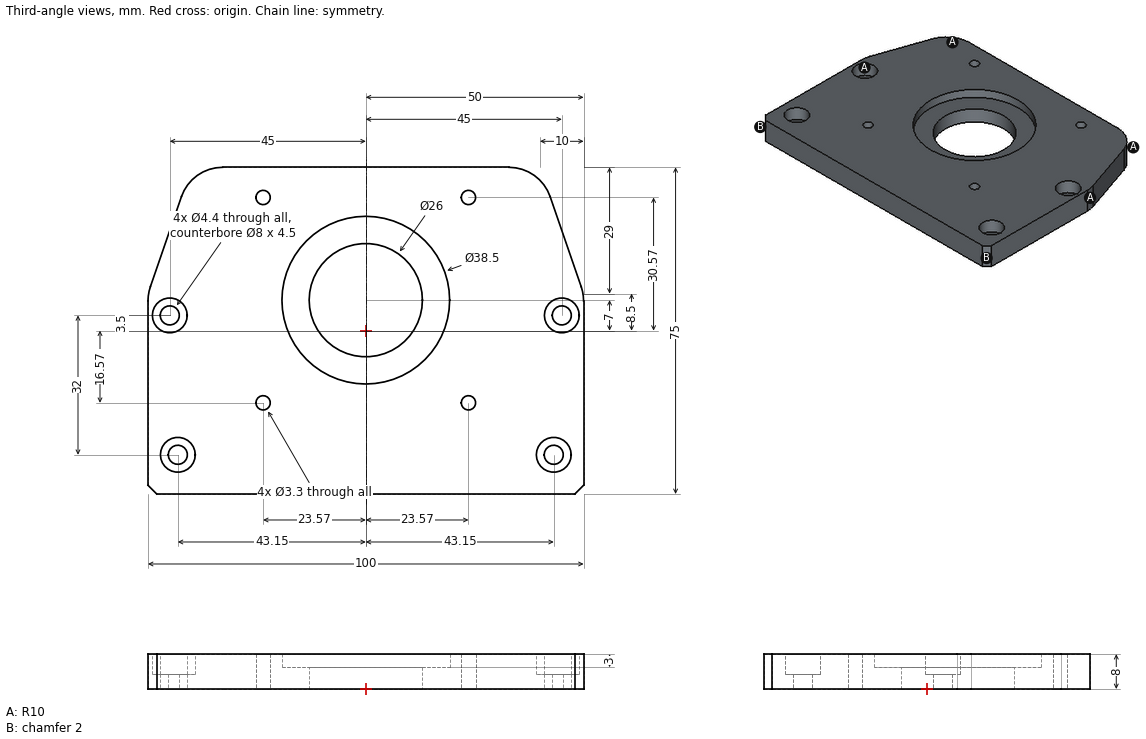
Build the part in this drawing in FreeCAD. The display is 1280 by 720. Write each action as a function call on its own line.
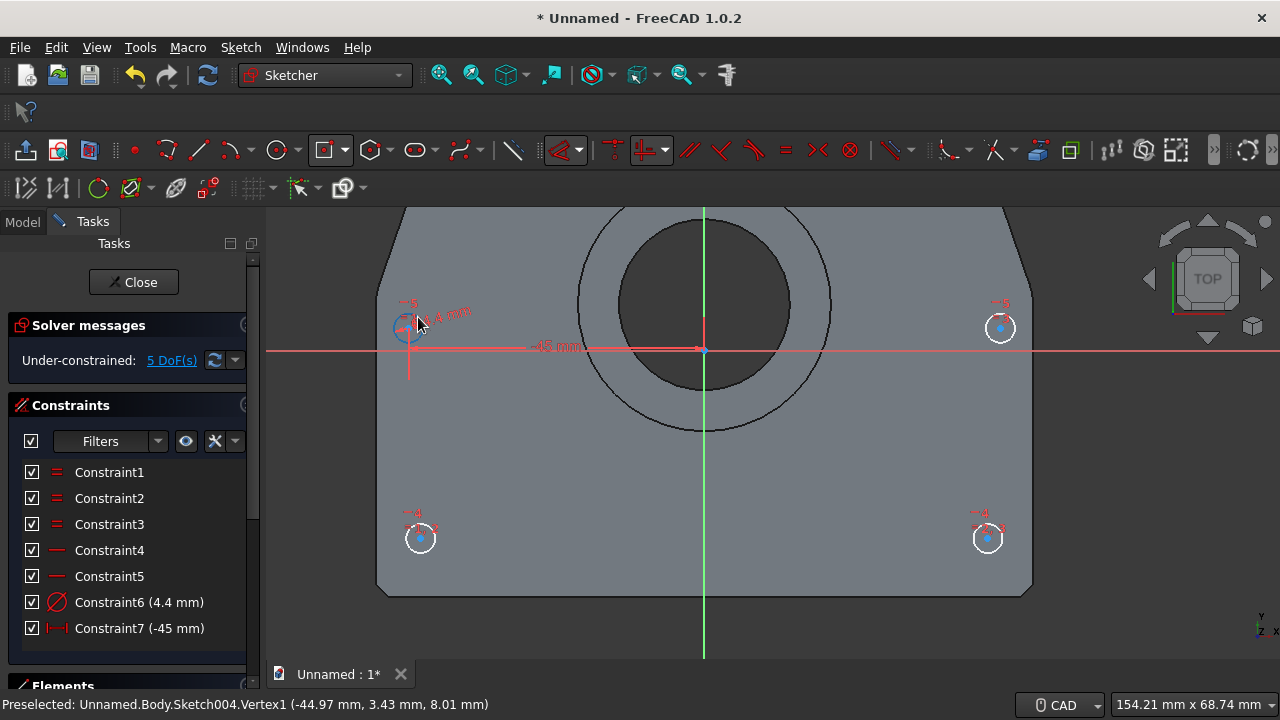
click(1000, 328)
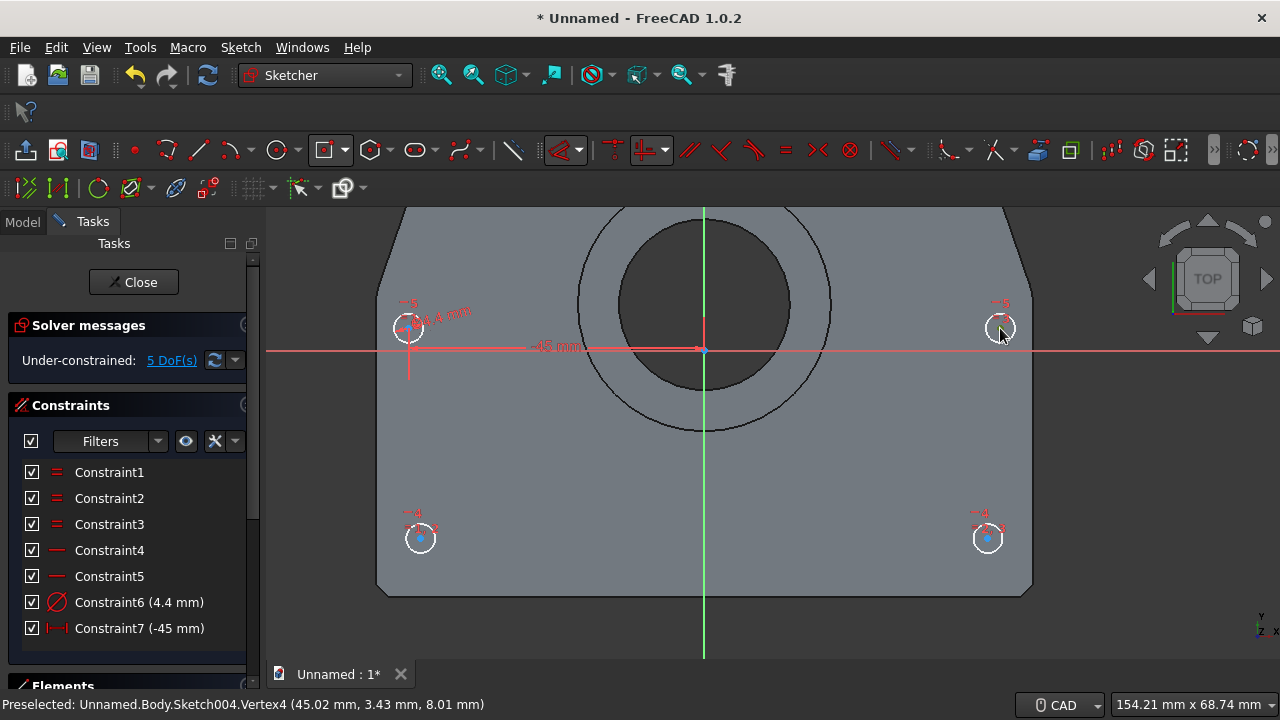
click(582, 150)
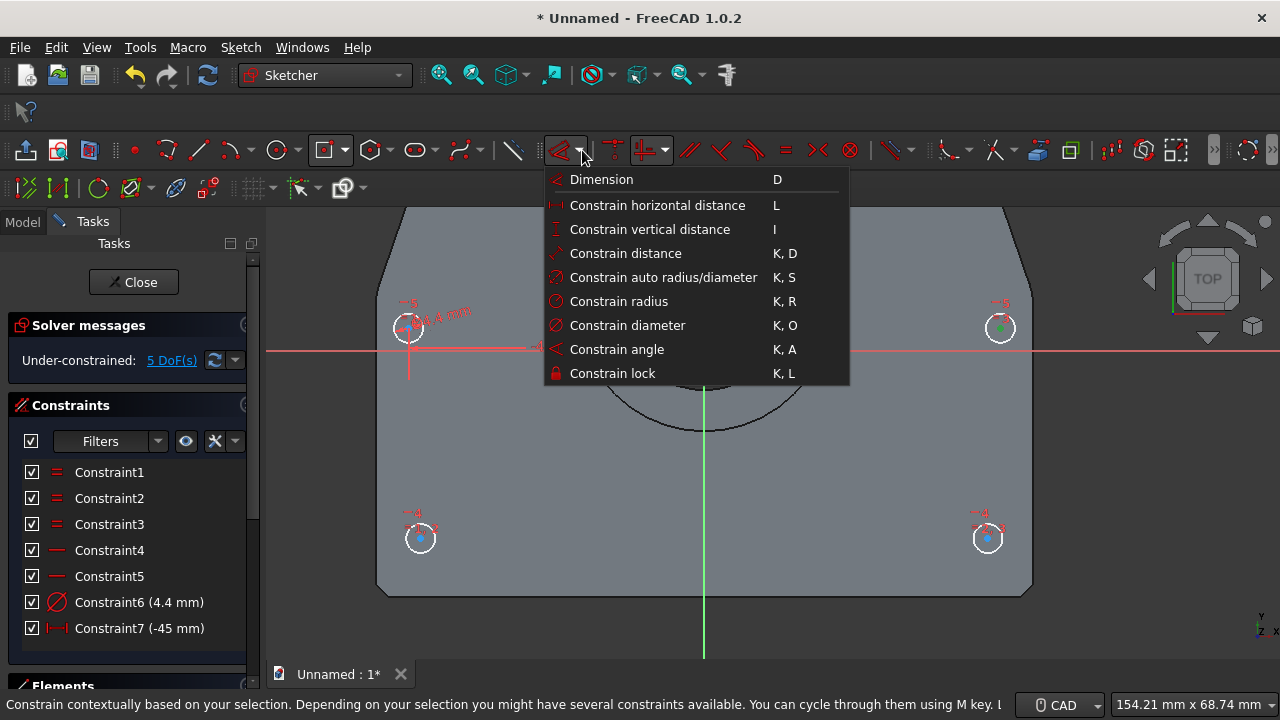
click(697, 205)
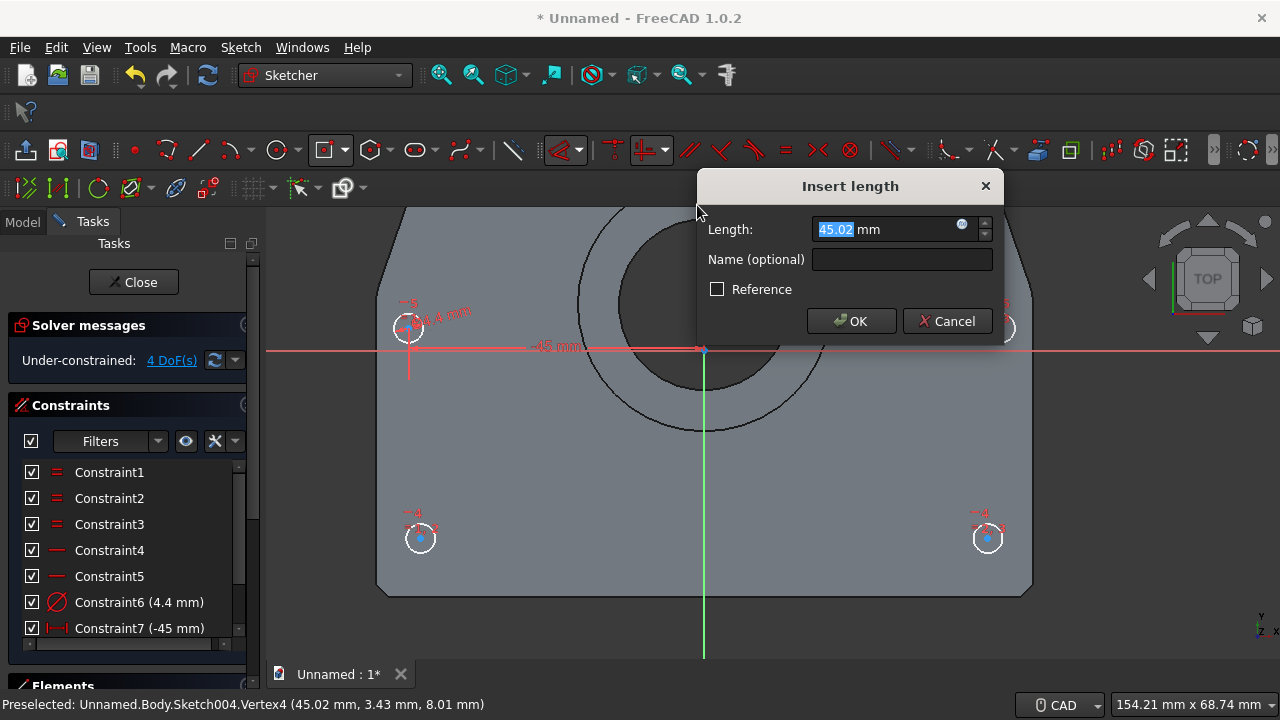
text(45)
key(Return)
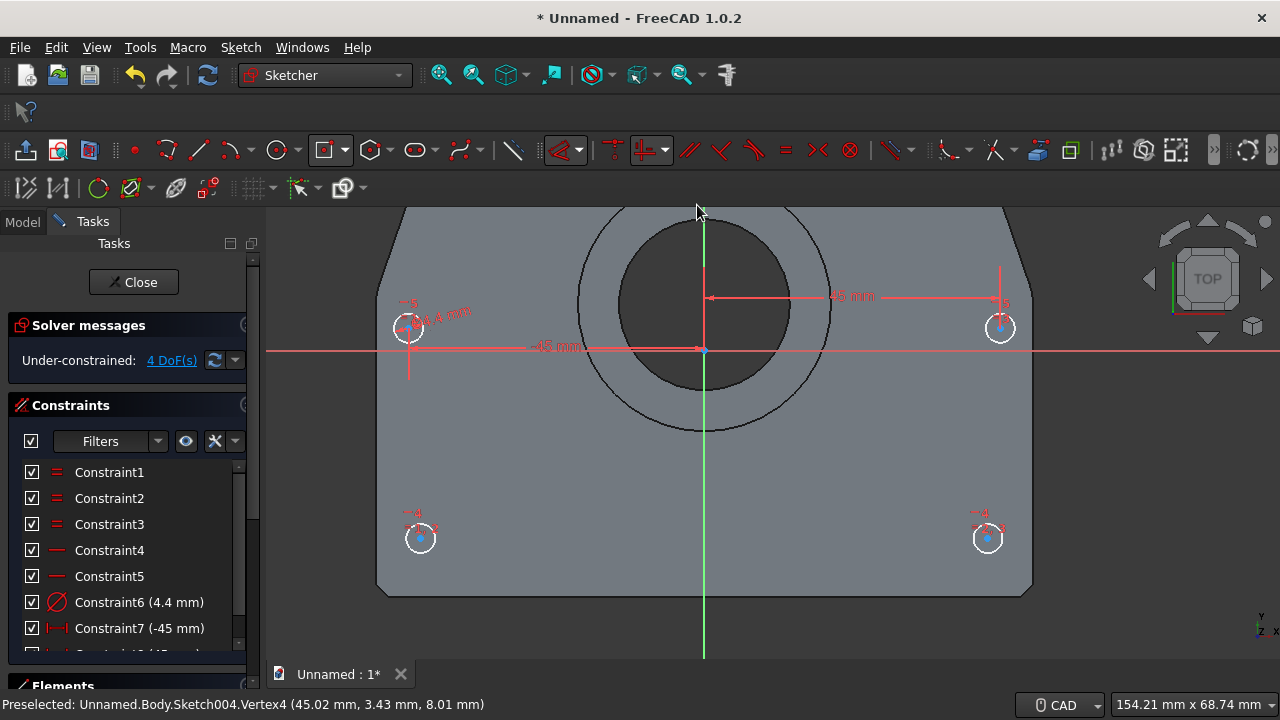
scroll(409, 328, up, 3)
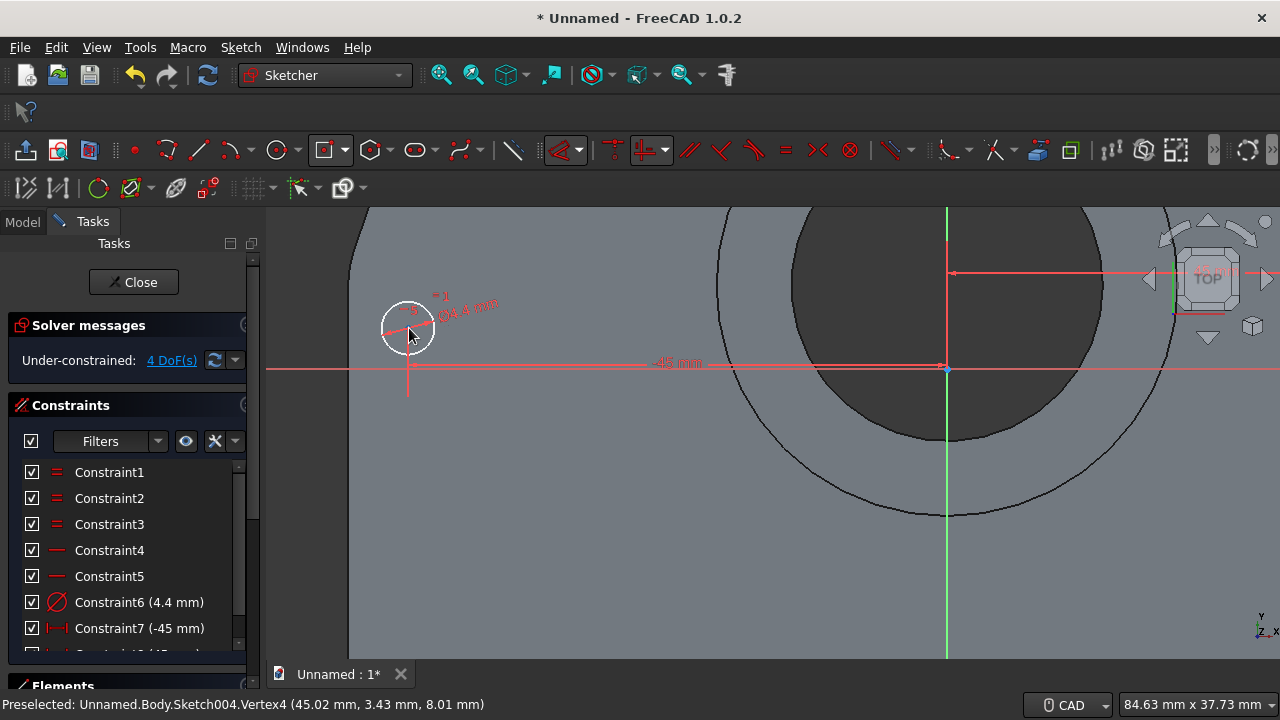
click(408, 328)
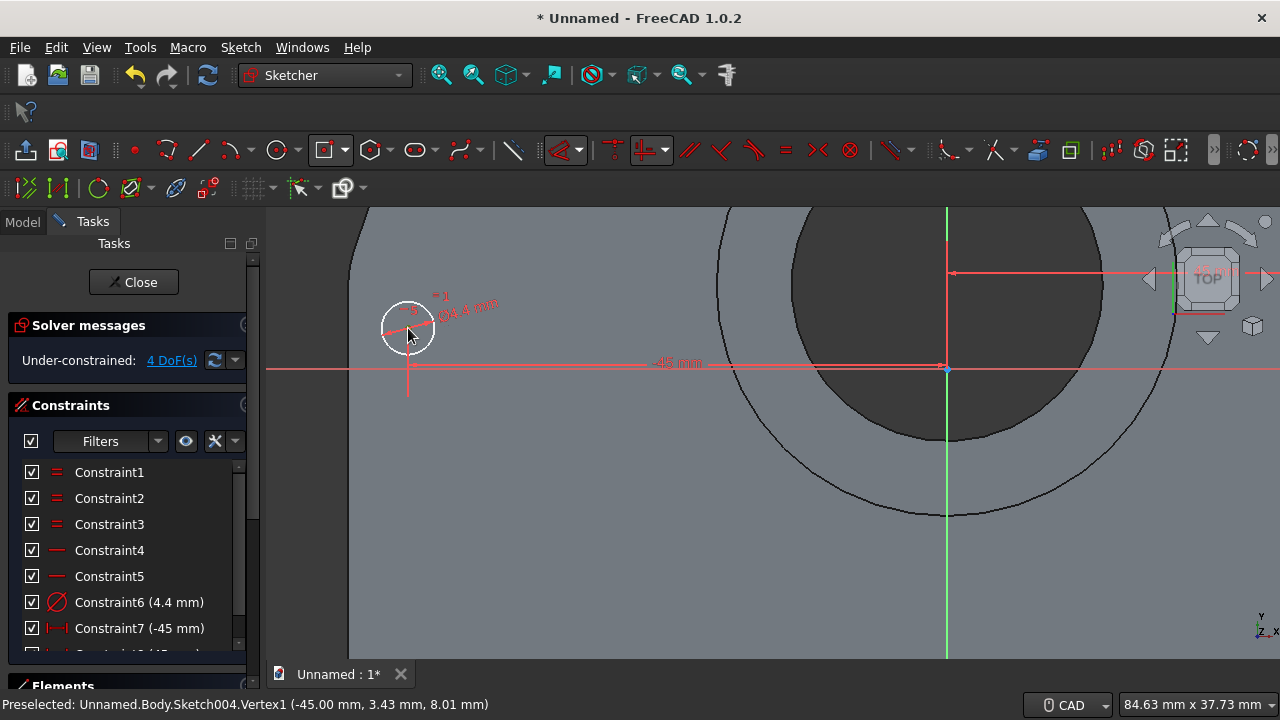
click(582, 150)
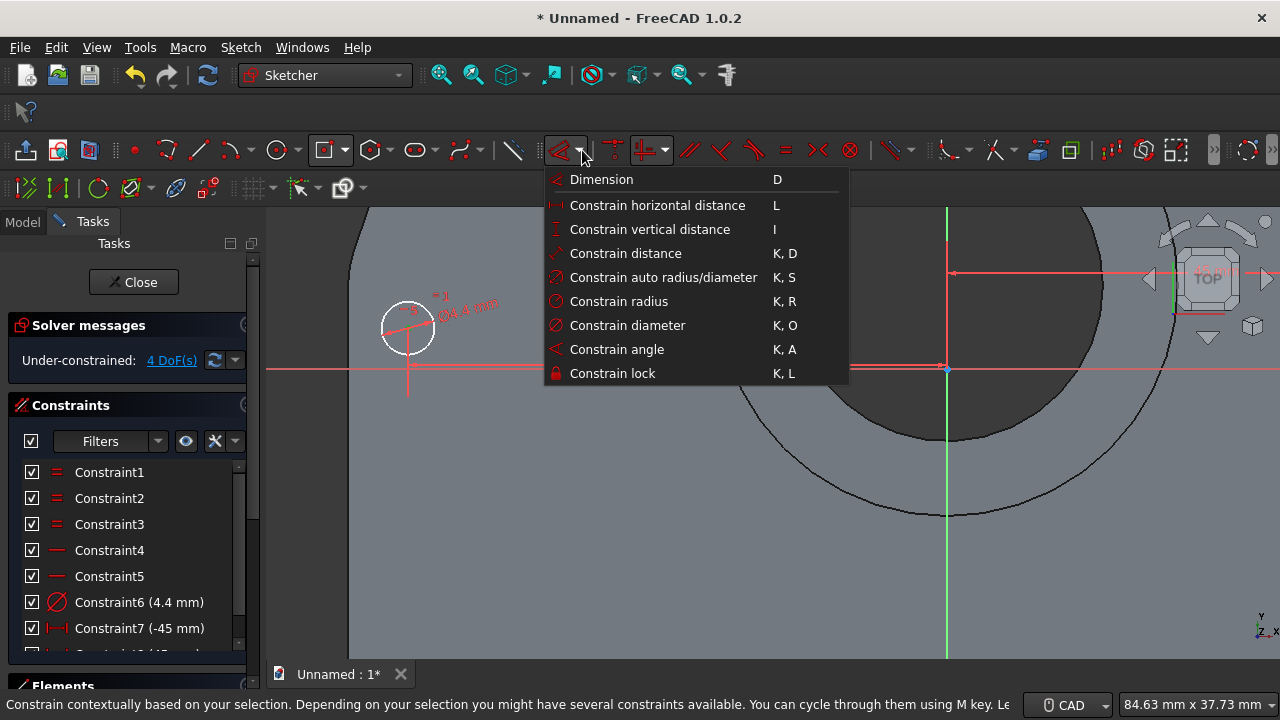
click(697, 229)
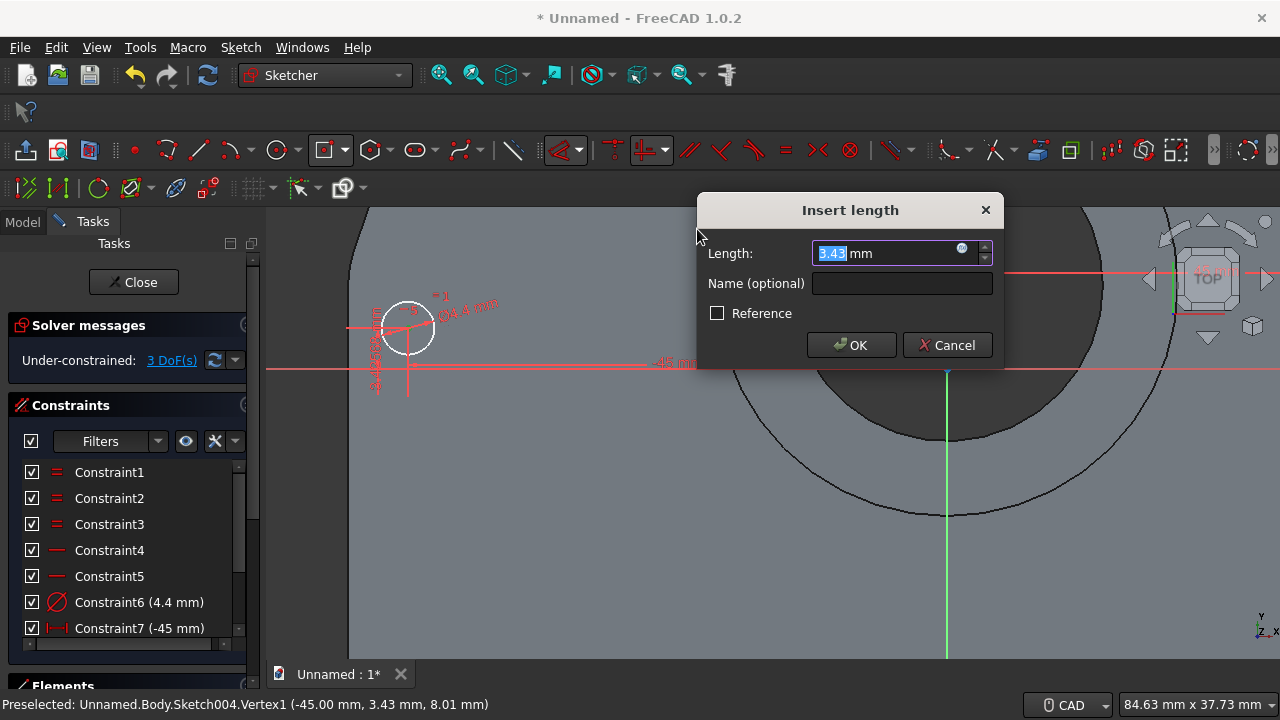
text(3.5)
key(Return)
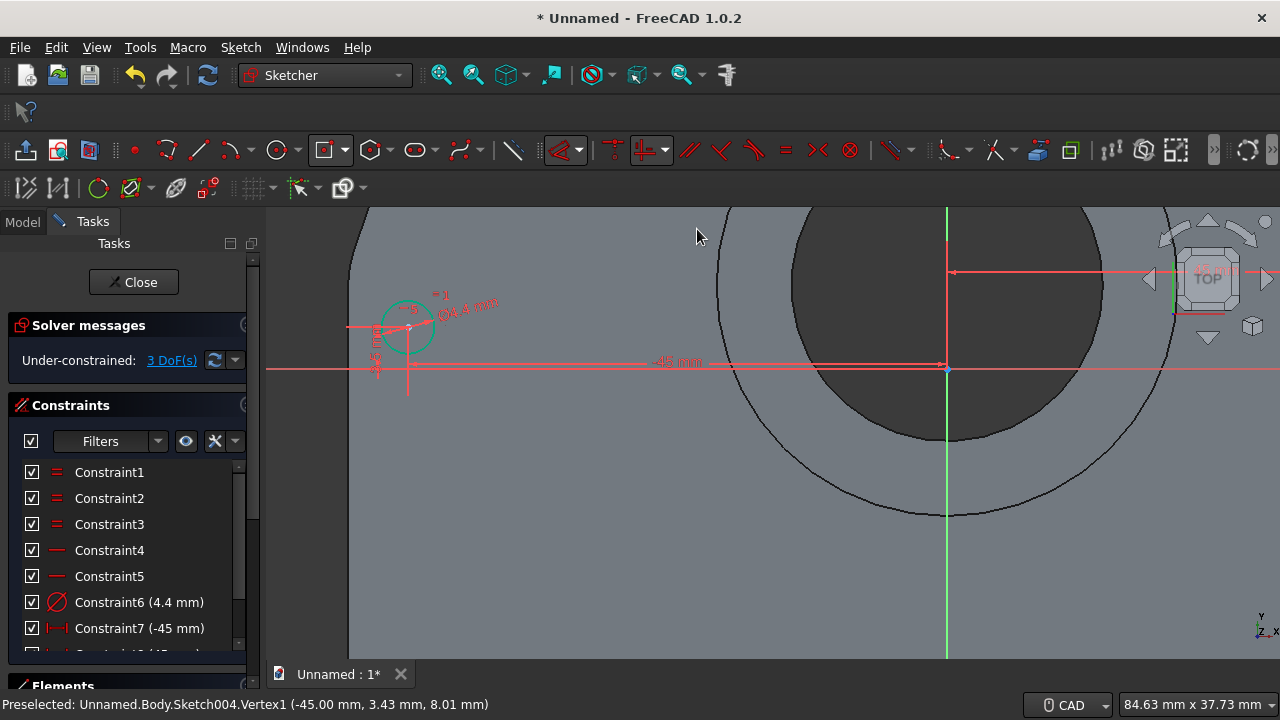
click(408, 327)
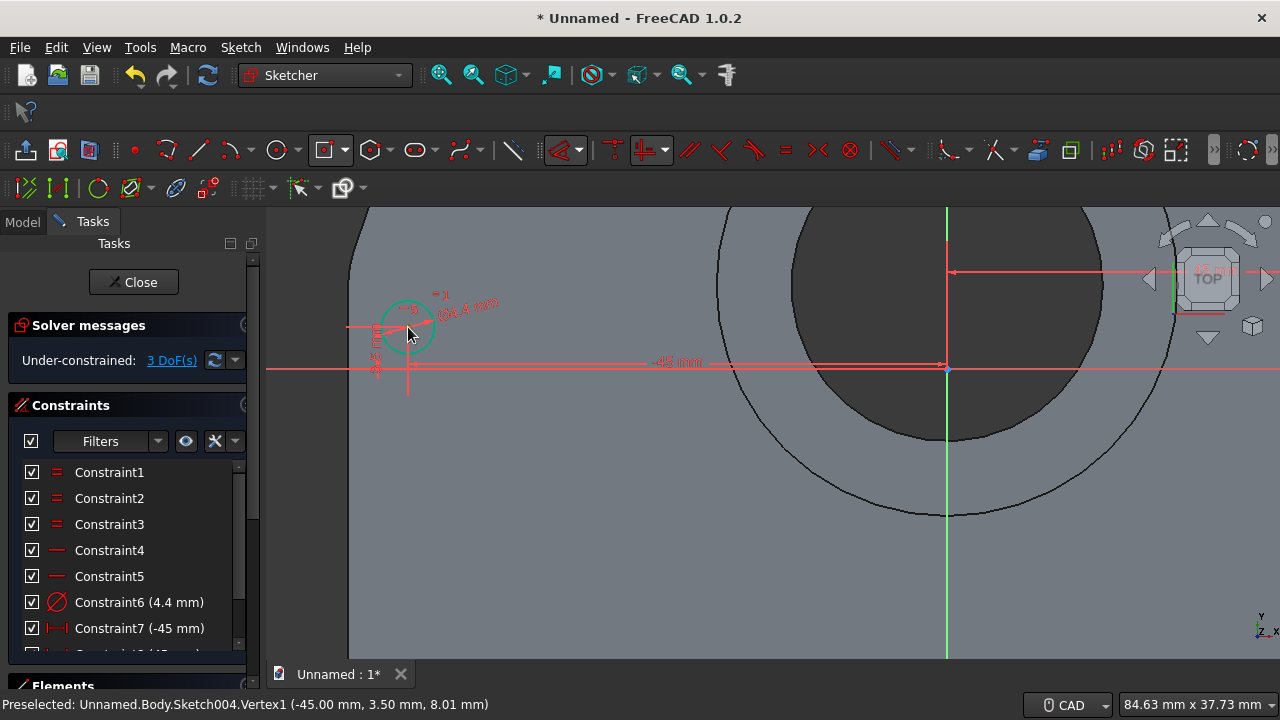
scroll(409, 328, down, 3)